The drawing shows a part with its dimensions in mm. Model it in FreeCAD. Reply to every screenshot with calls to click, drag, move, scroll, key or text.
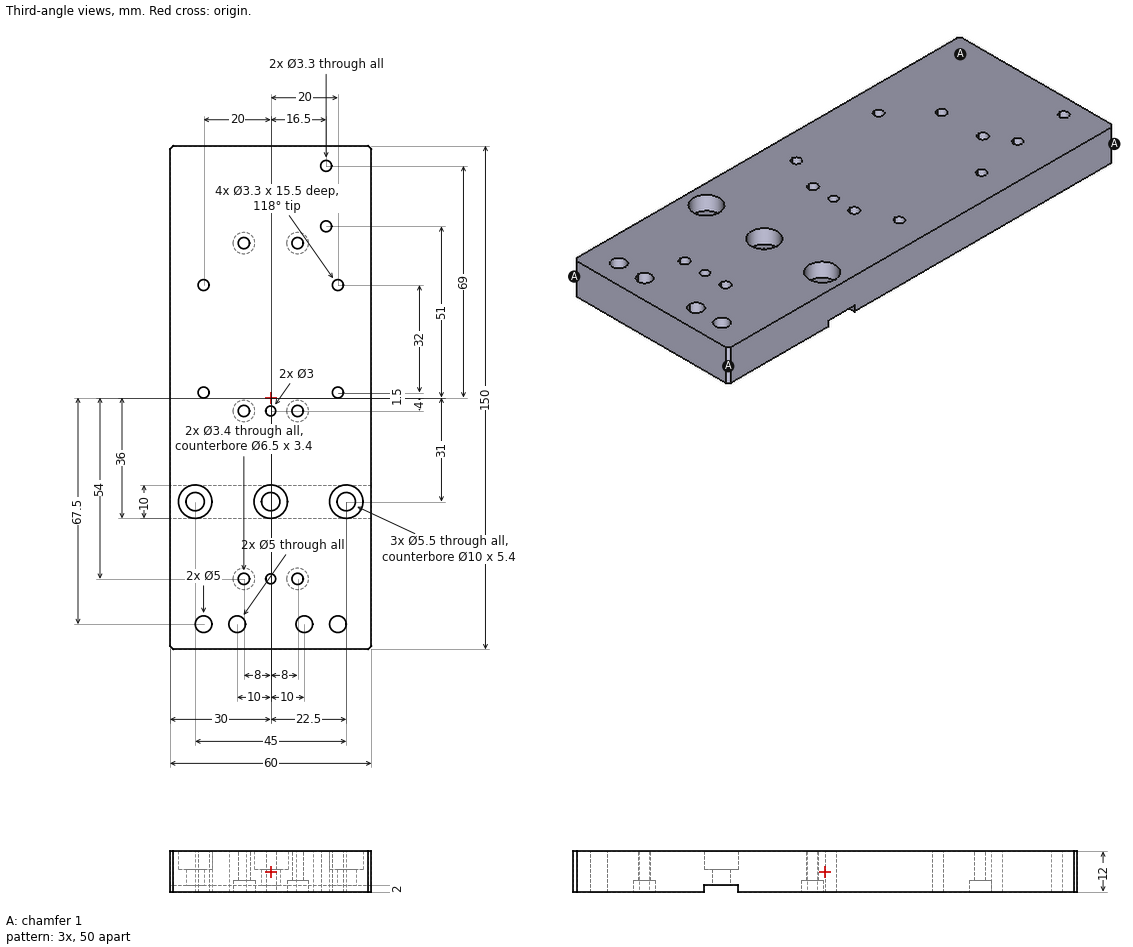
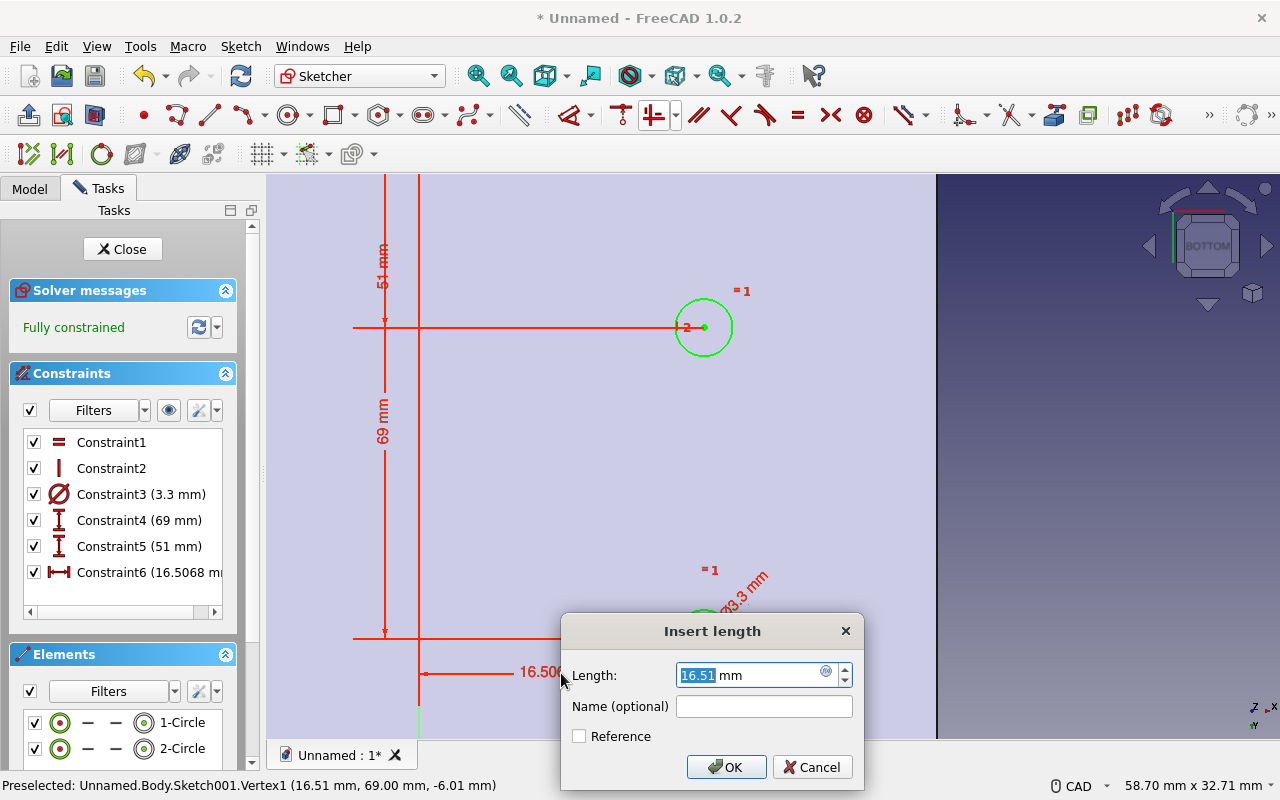
text(16.5)
key(Return)
key(Escape)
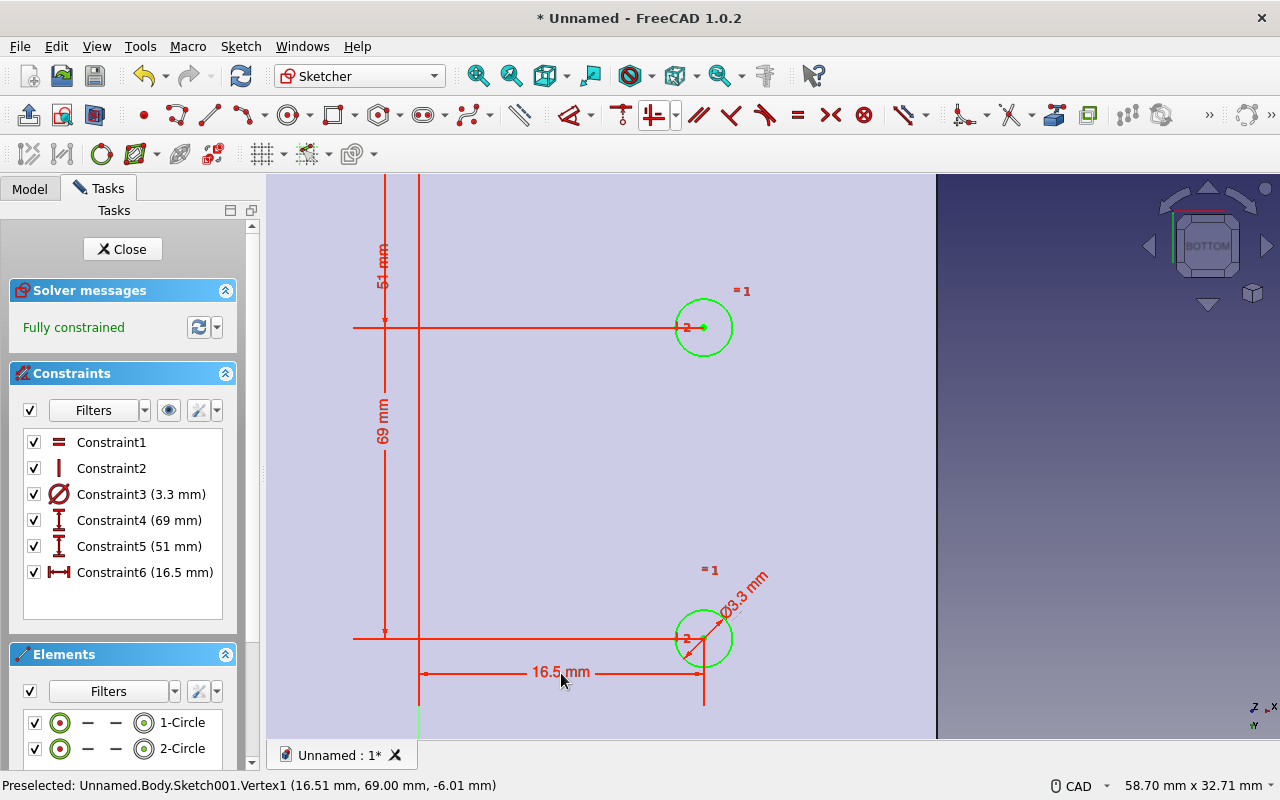
click(123, 249)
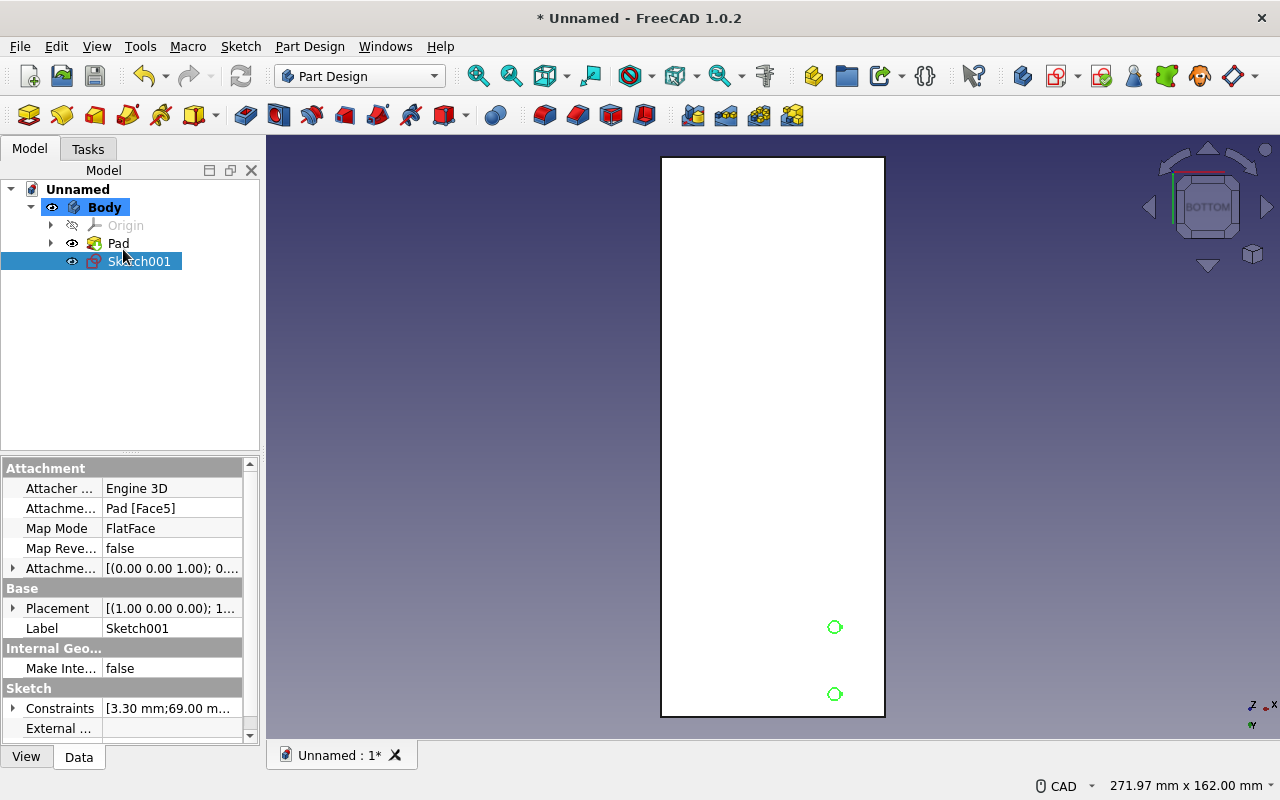
click(279, 116)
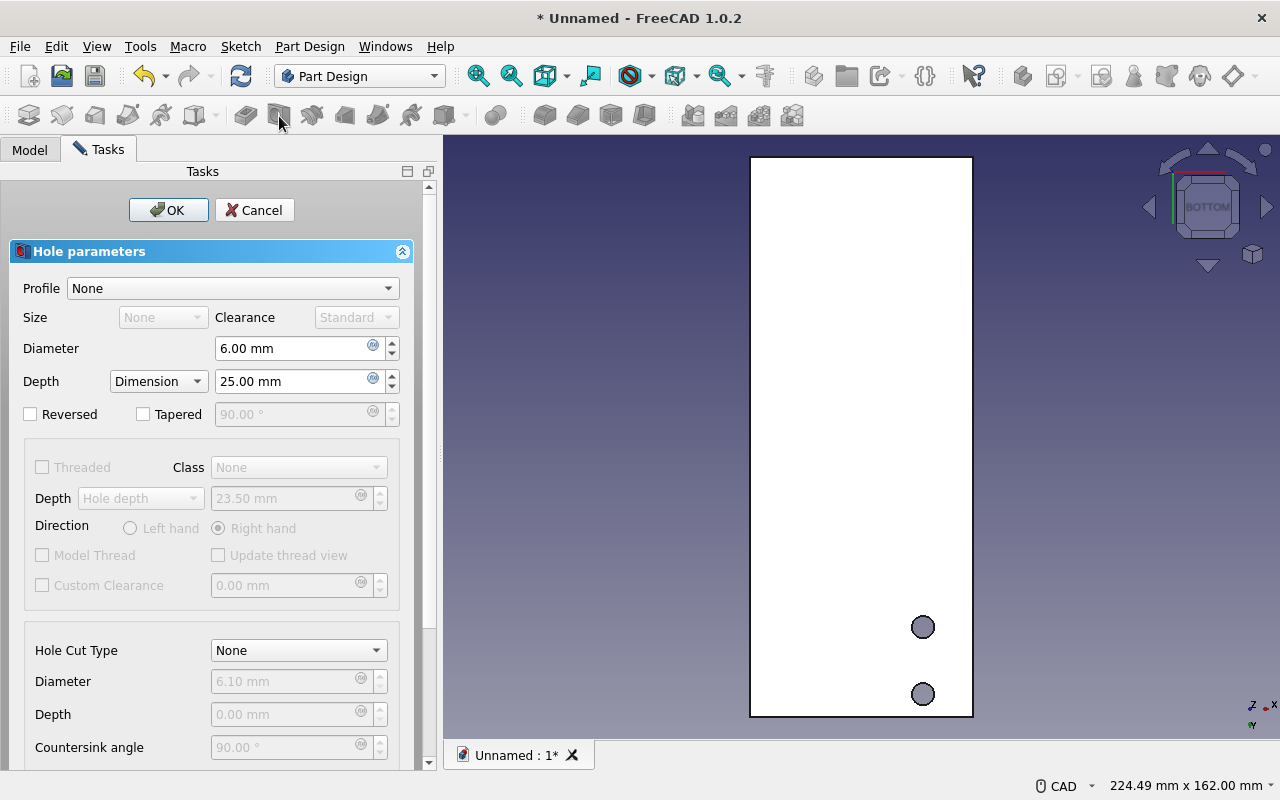
triple_click(300, 348)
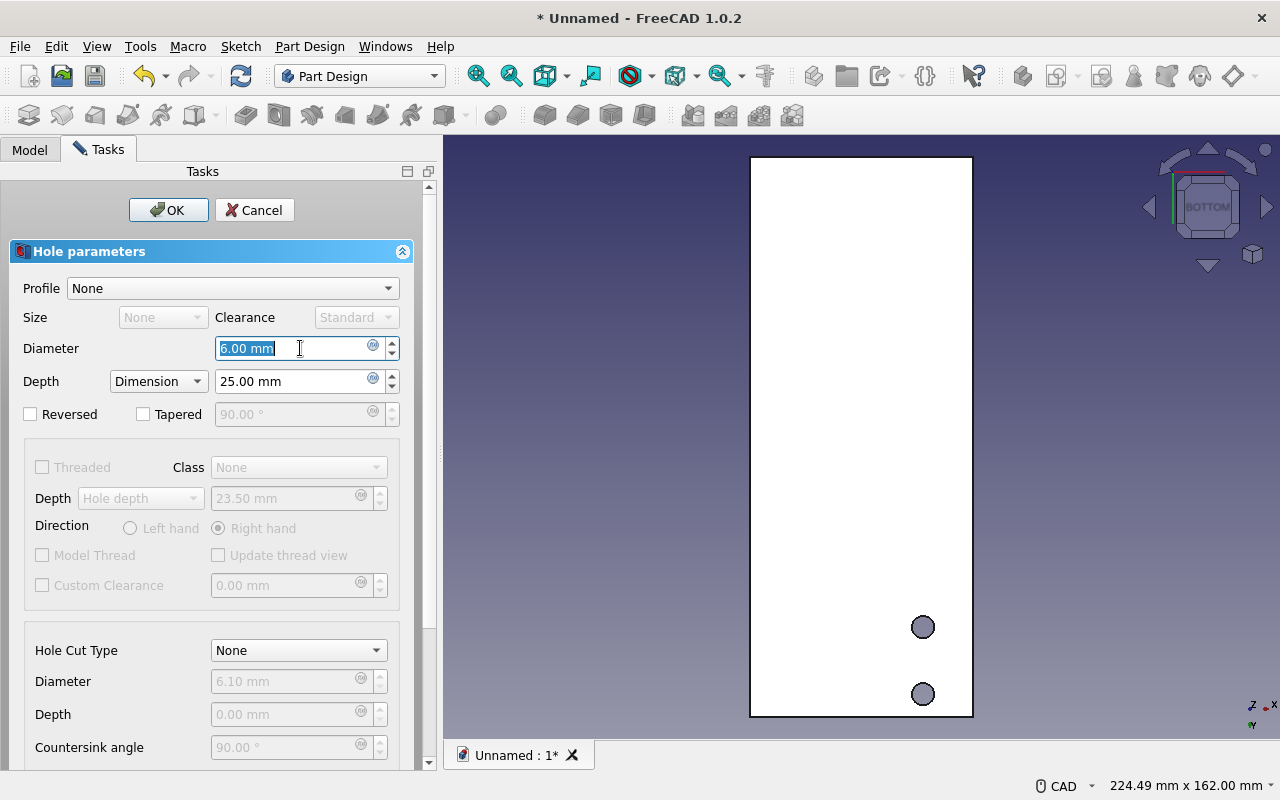
text(3.3)
key(Tab)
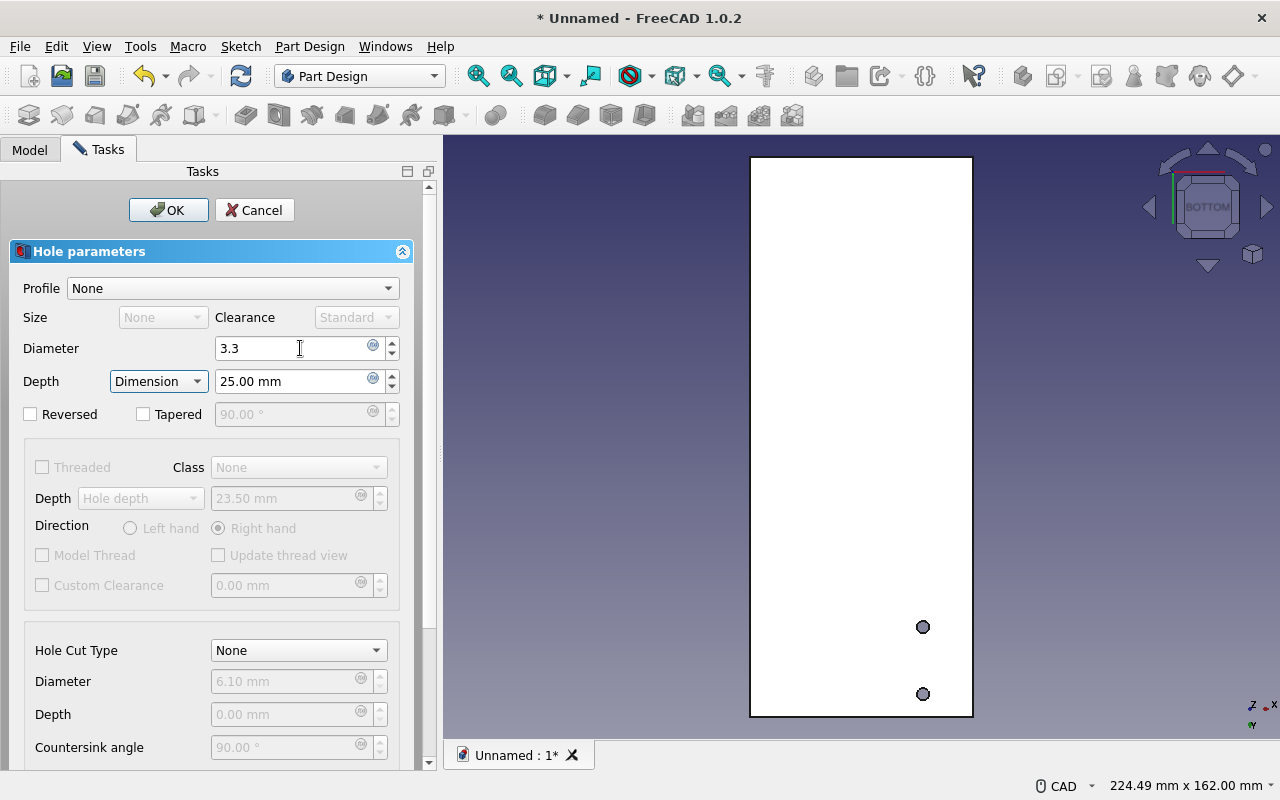
click(160, 382)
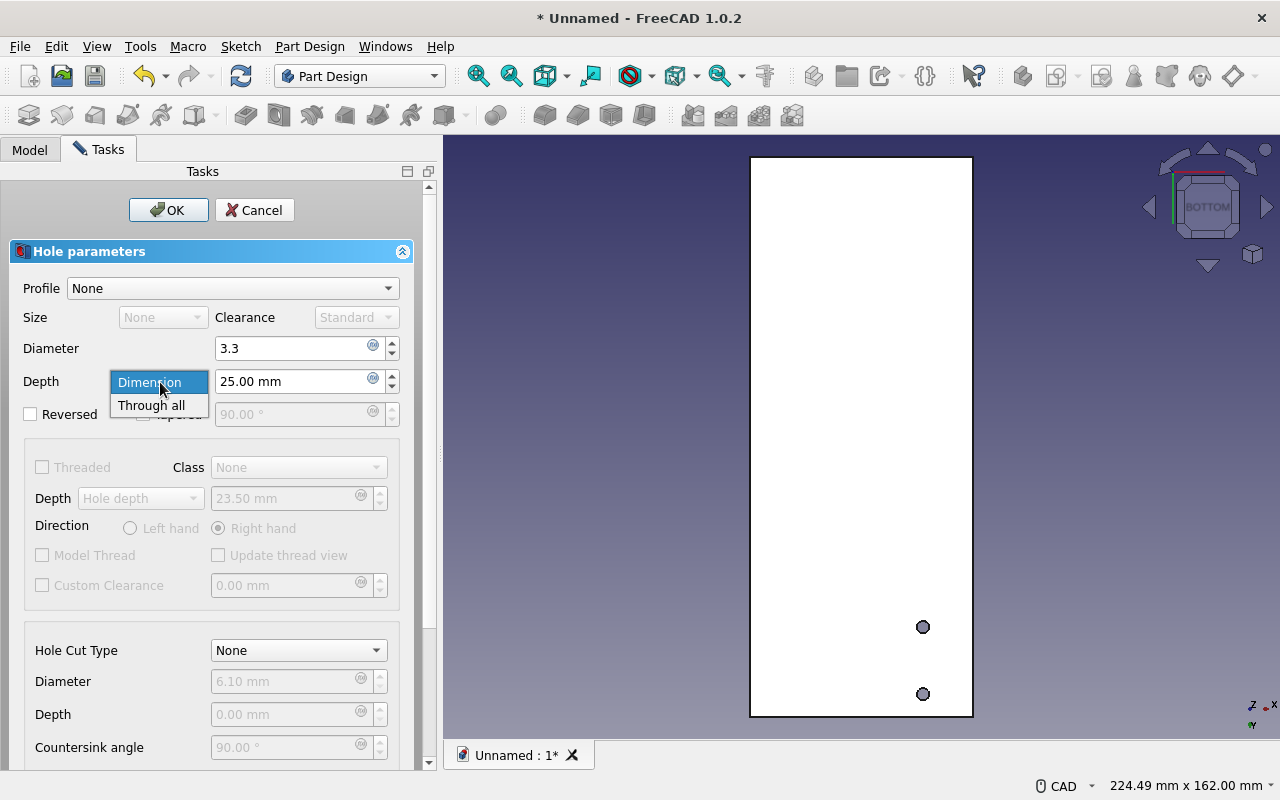
click(158, 406)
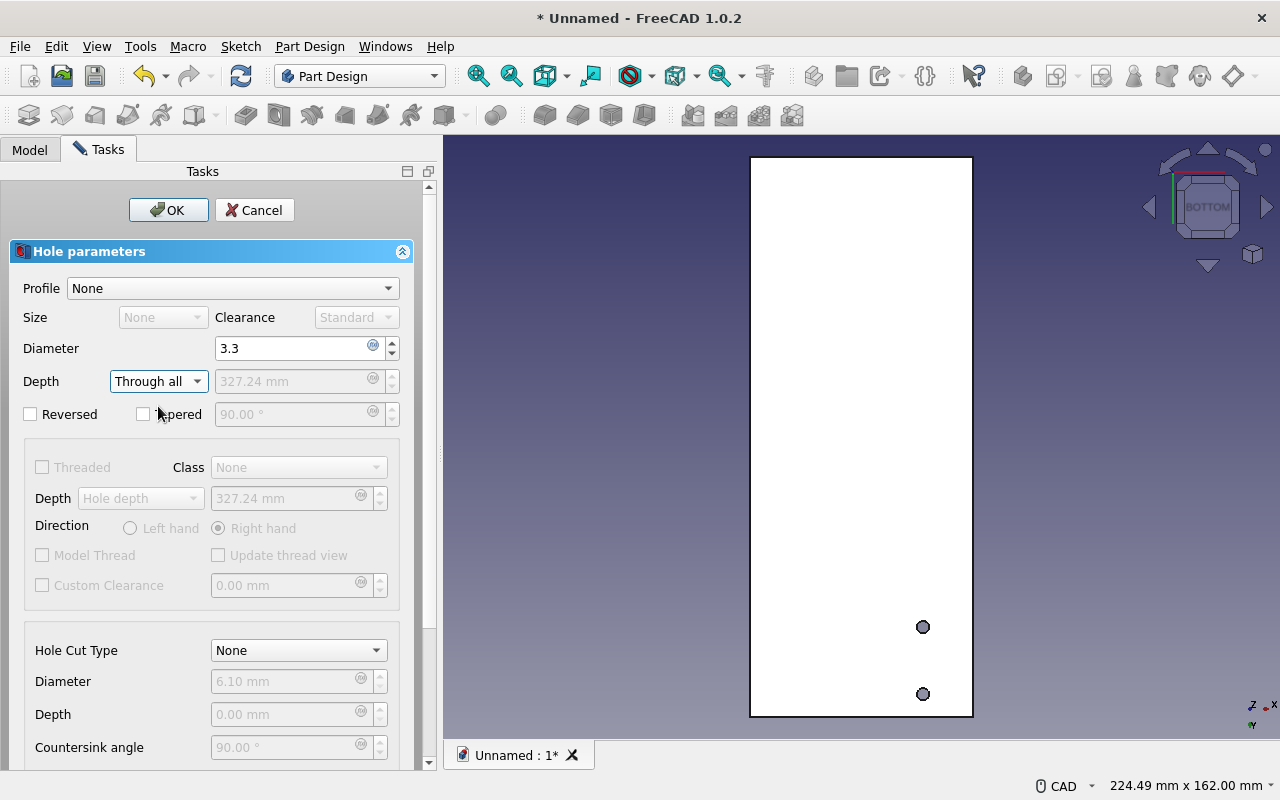
click(169, 210)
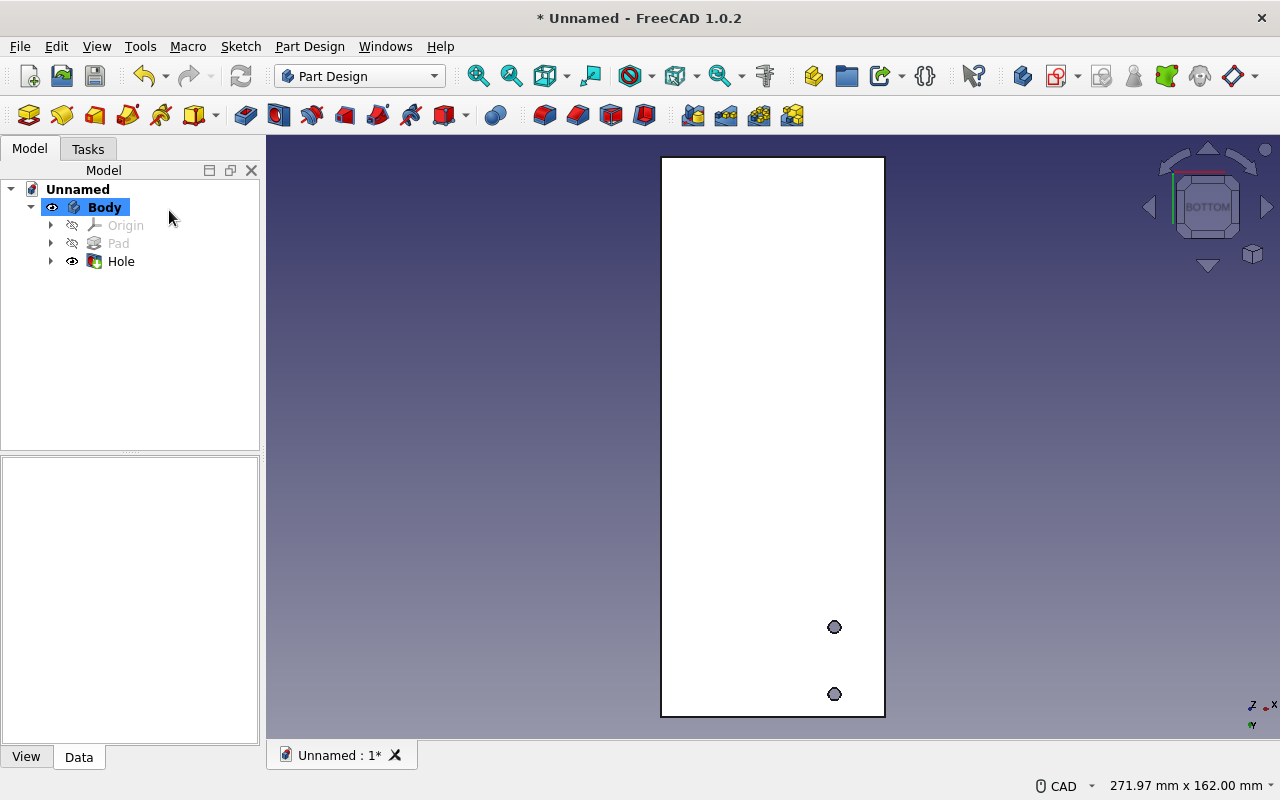
click(773, 516)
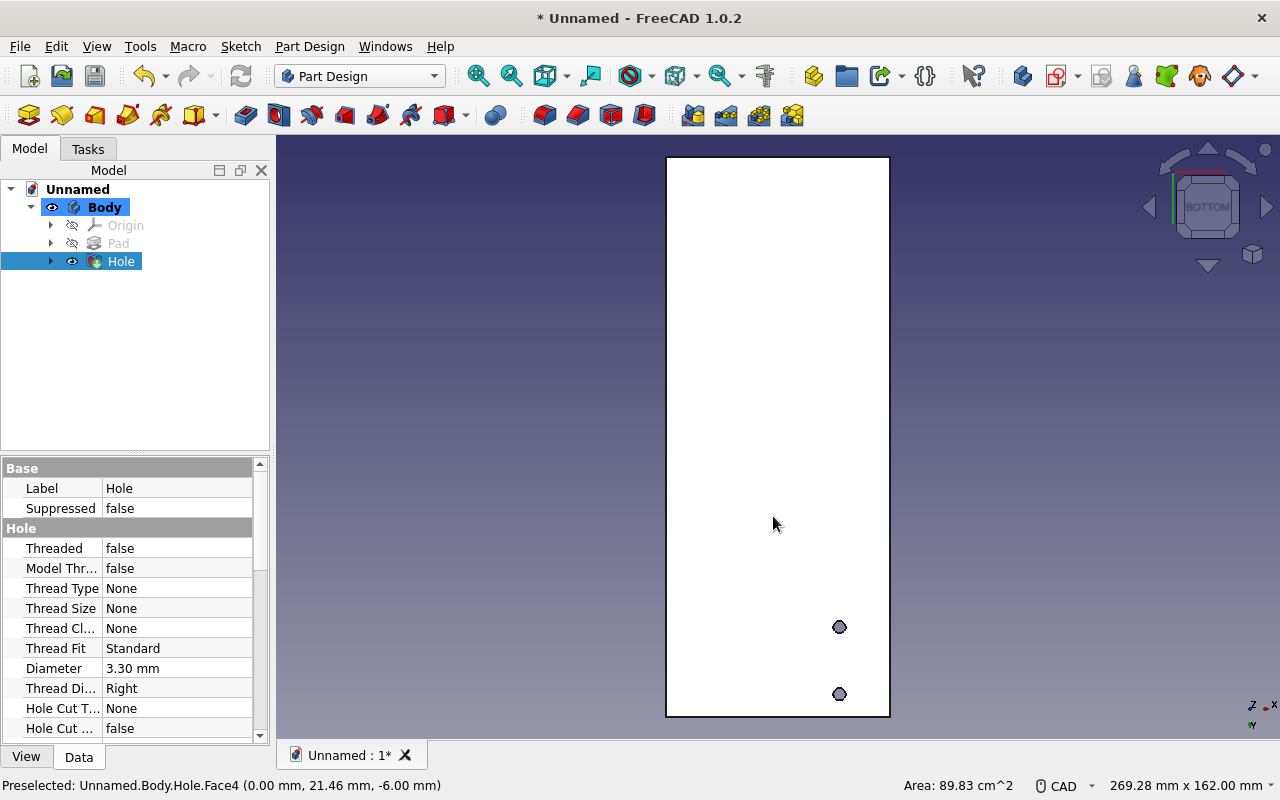
click(1056, 76)